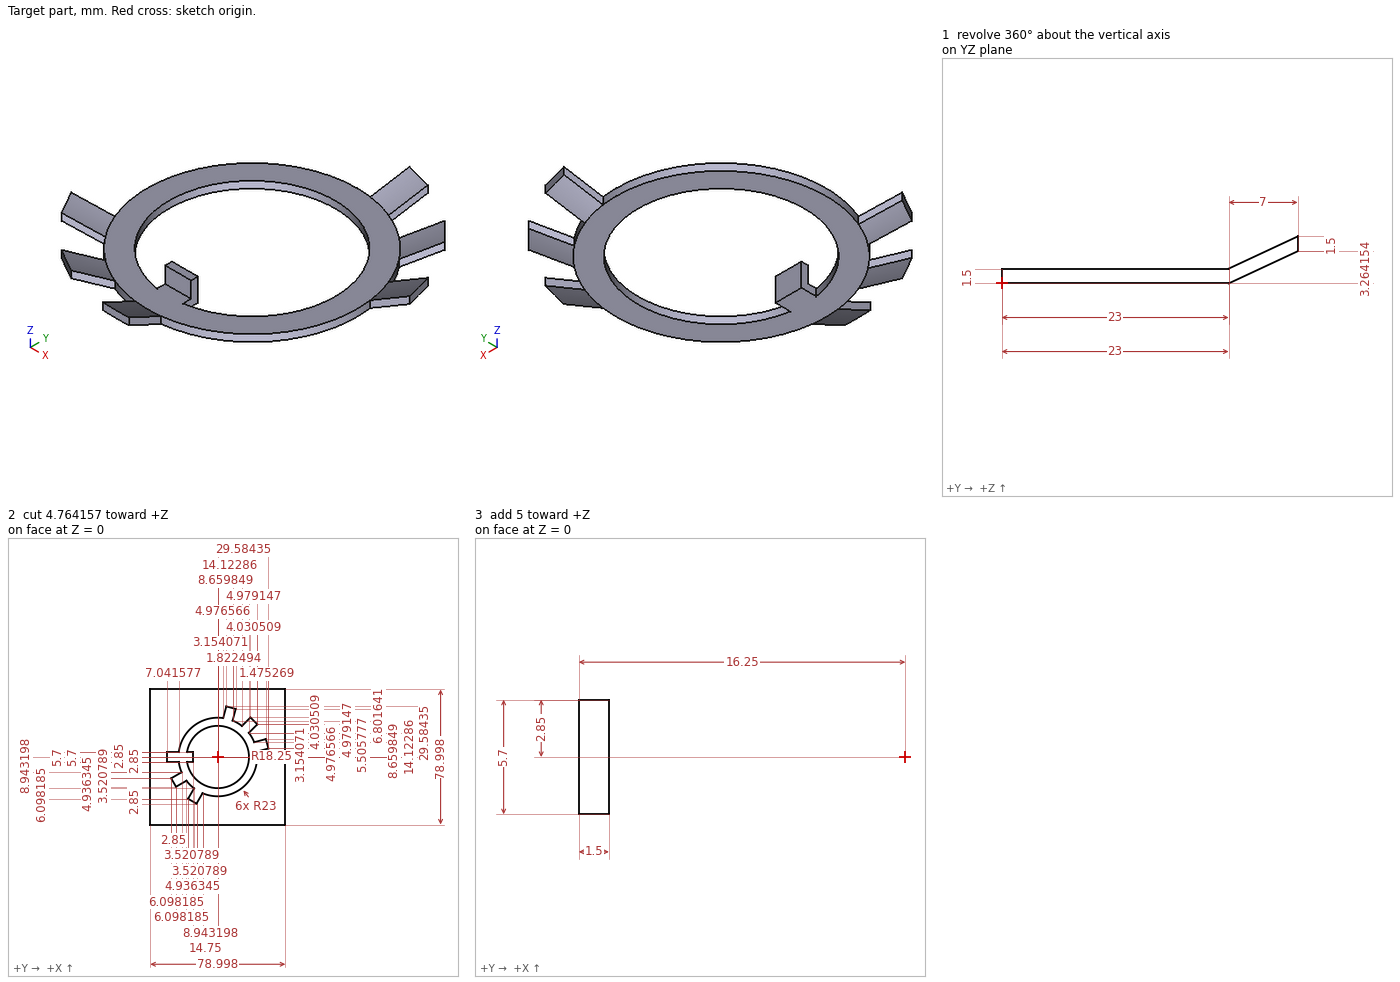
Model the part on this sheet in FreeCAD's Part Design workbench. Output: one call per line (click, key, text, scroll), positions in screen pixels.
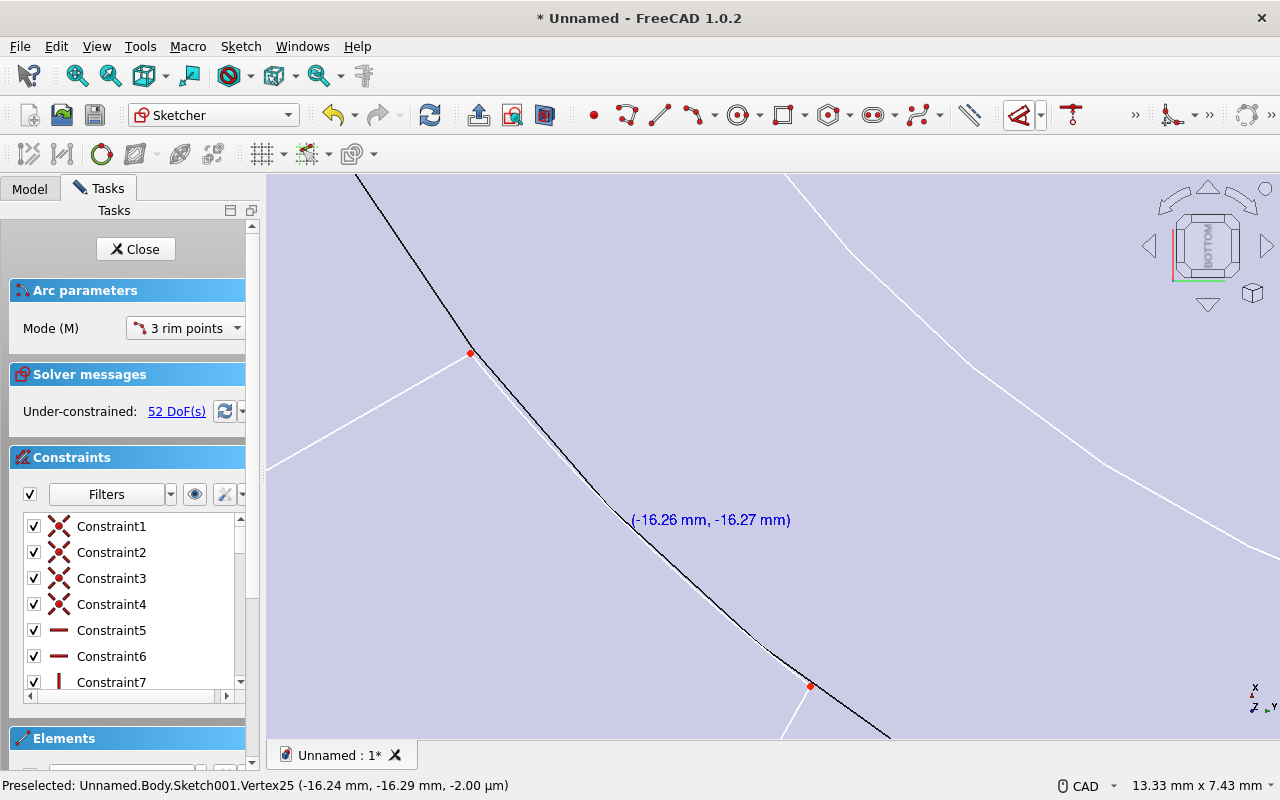
scroll(629, 532, down, 14)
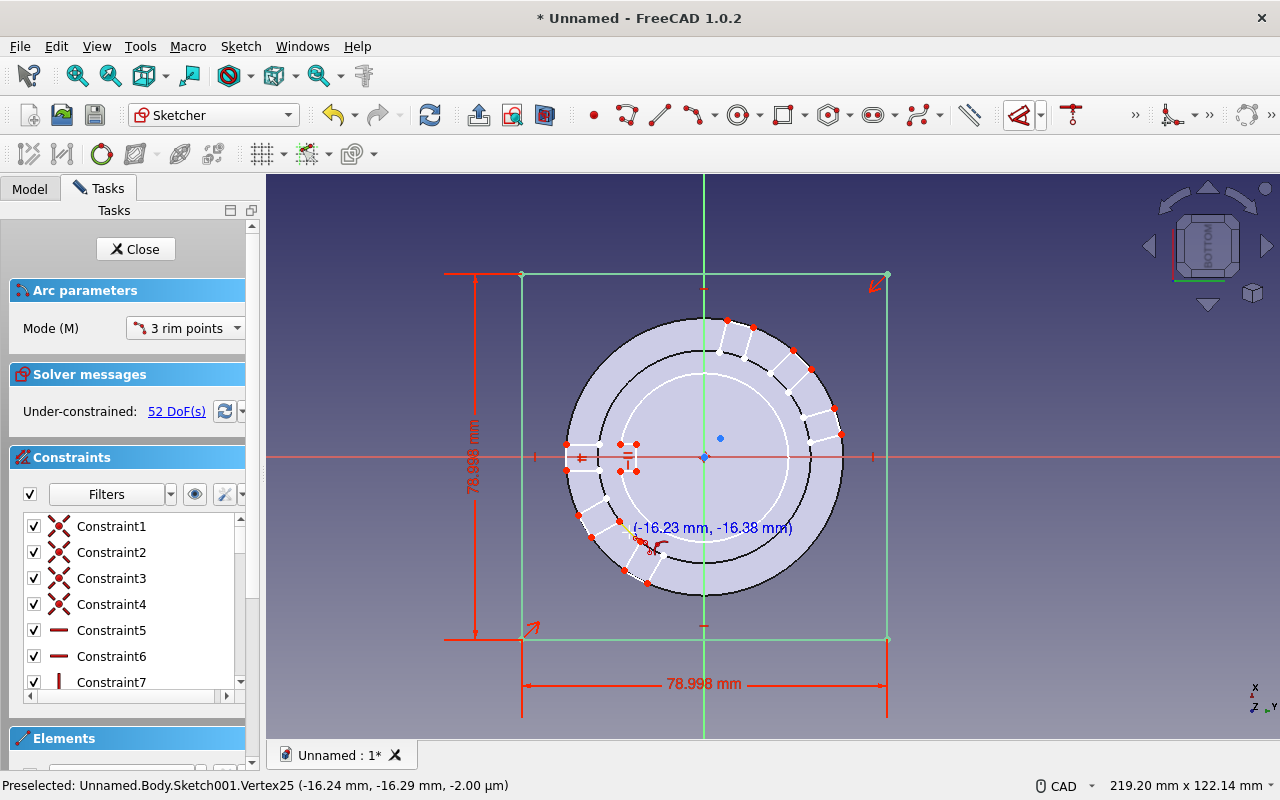
click(663, 556)
click(810, 443)
click(769, 541)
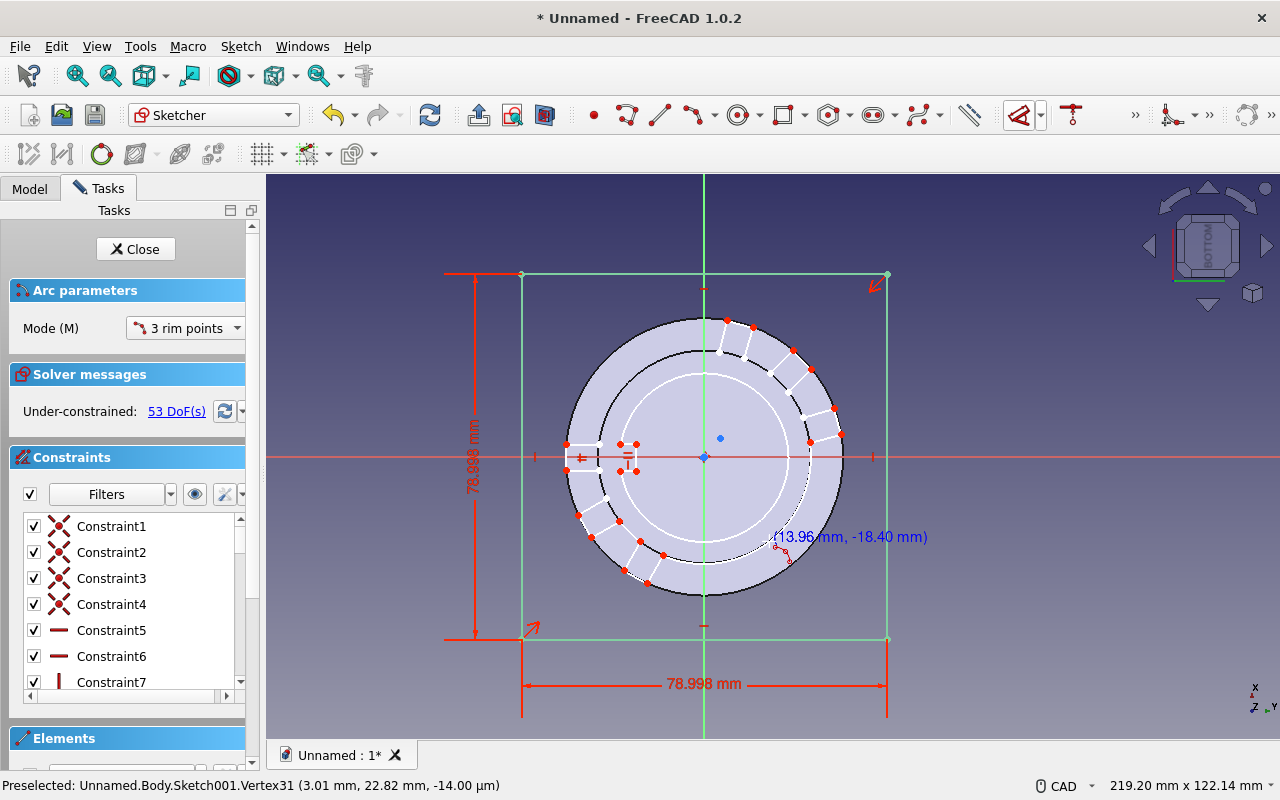
click(803, 418)
click(788, 393)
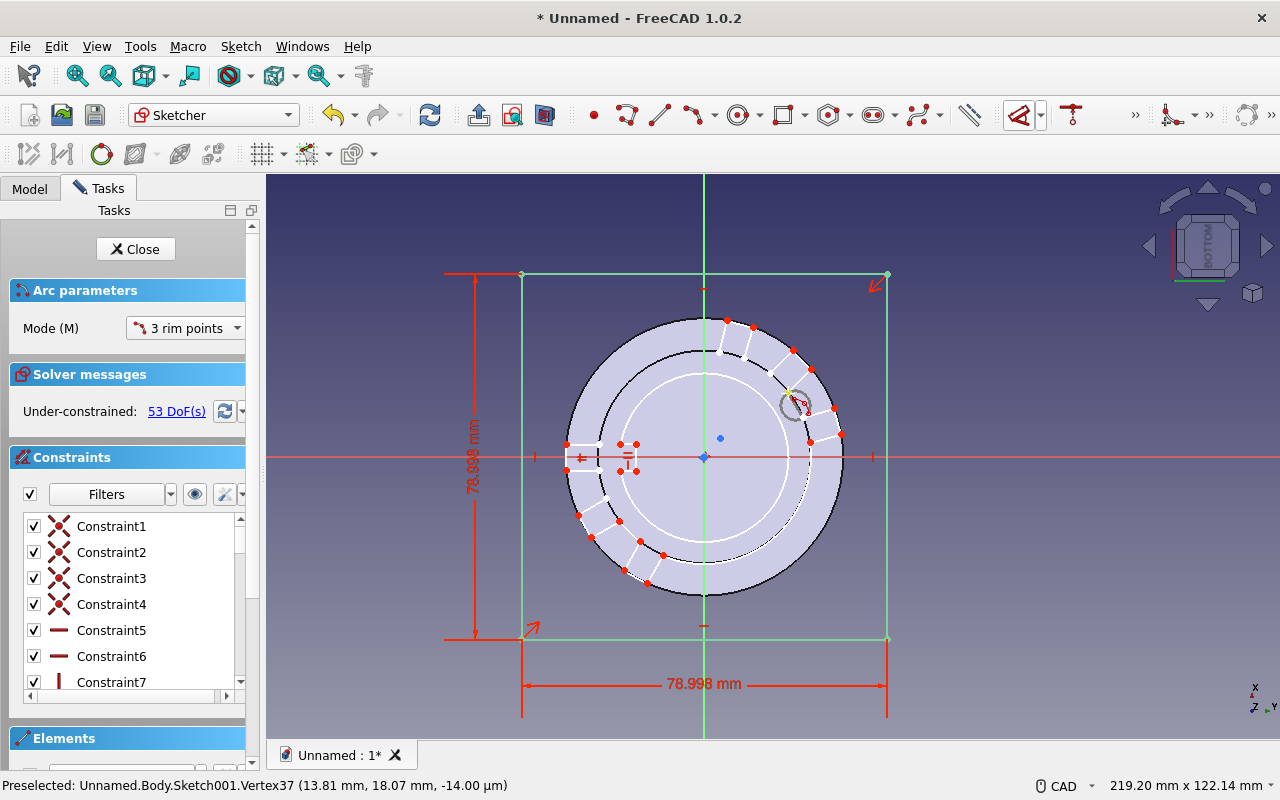
scroll(797, 404, up, 14)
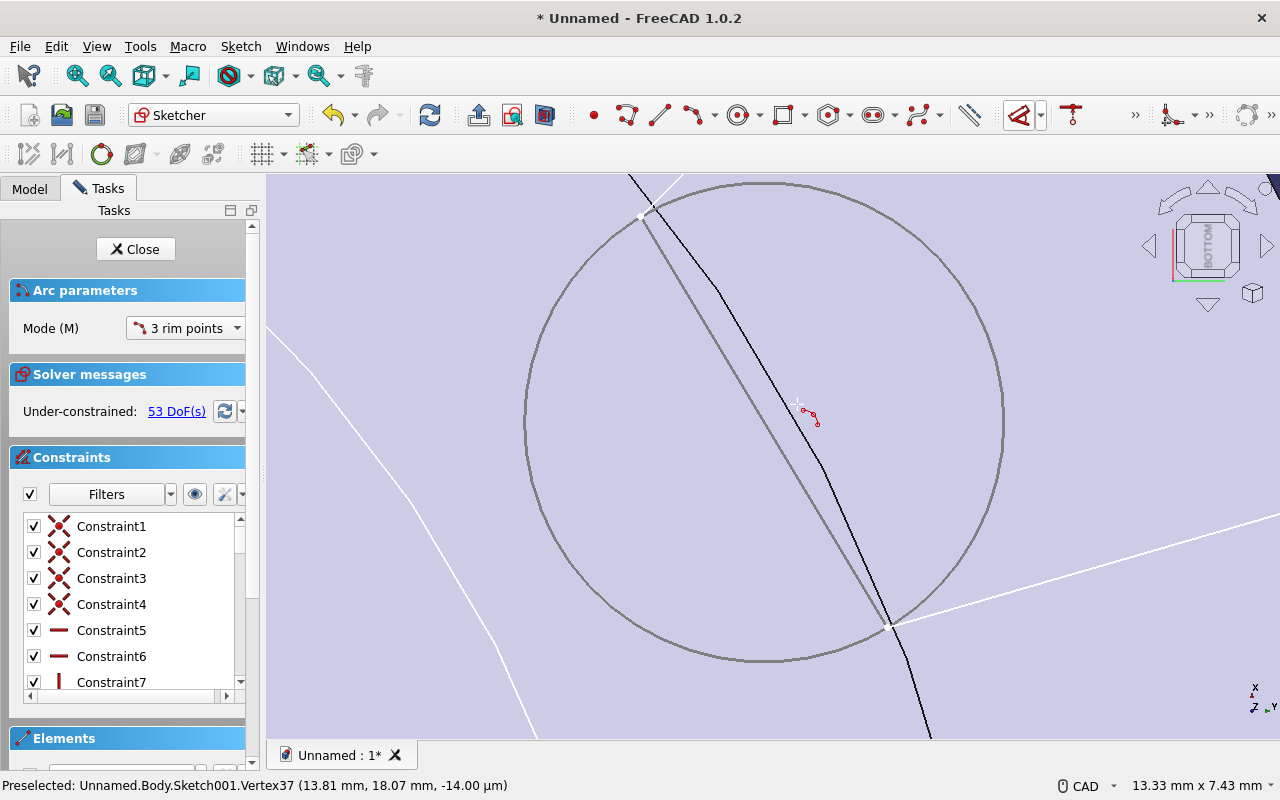
click(782, 393)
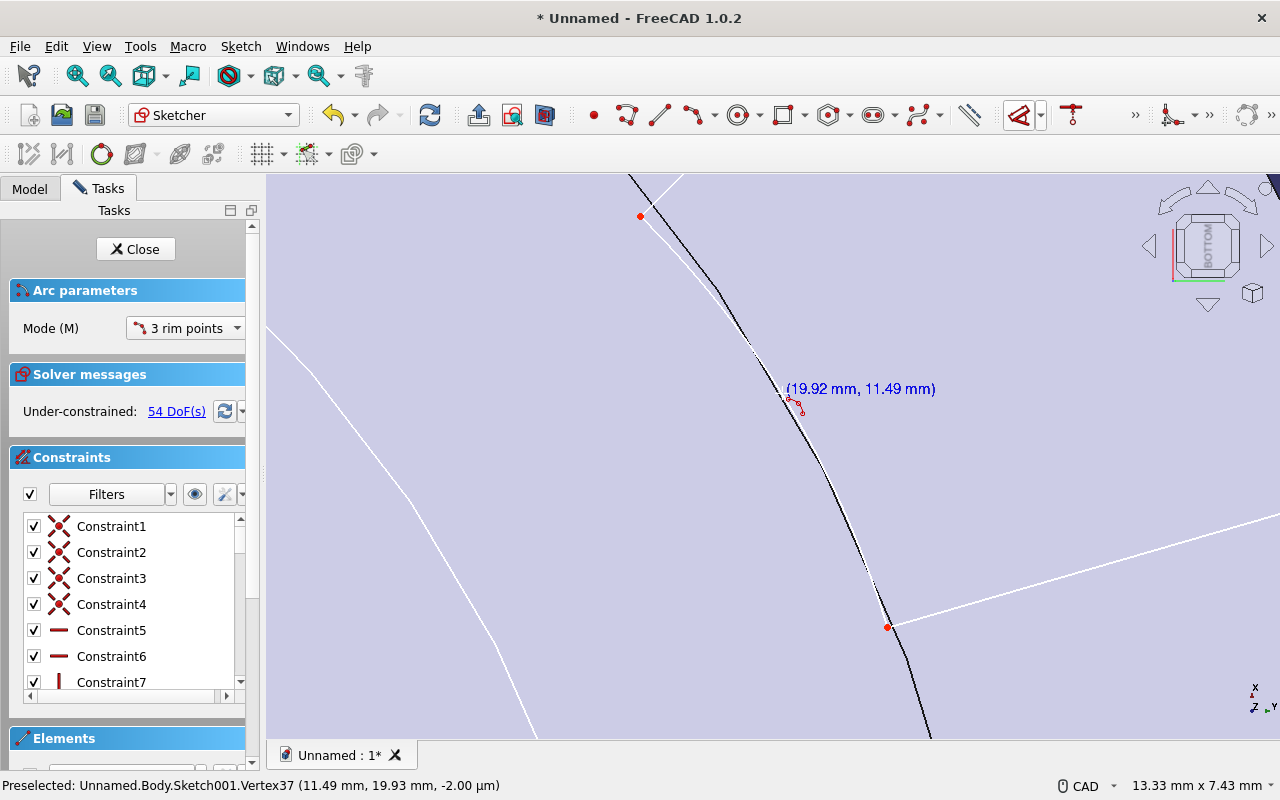
scroll(798, 404, down, 14)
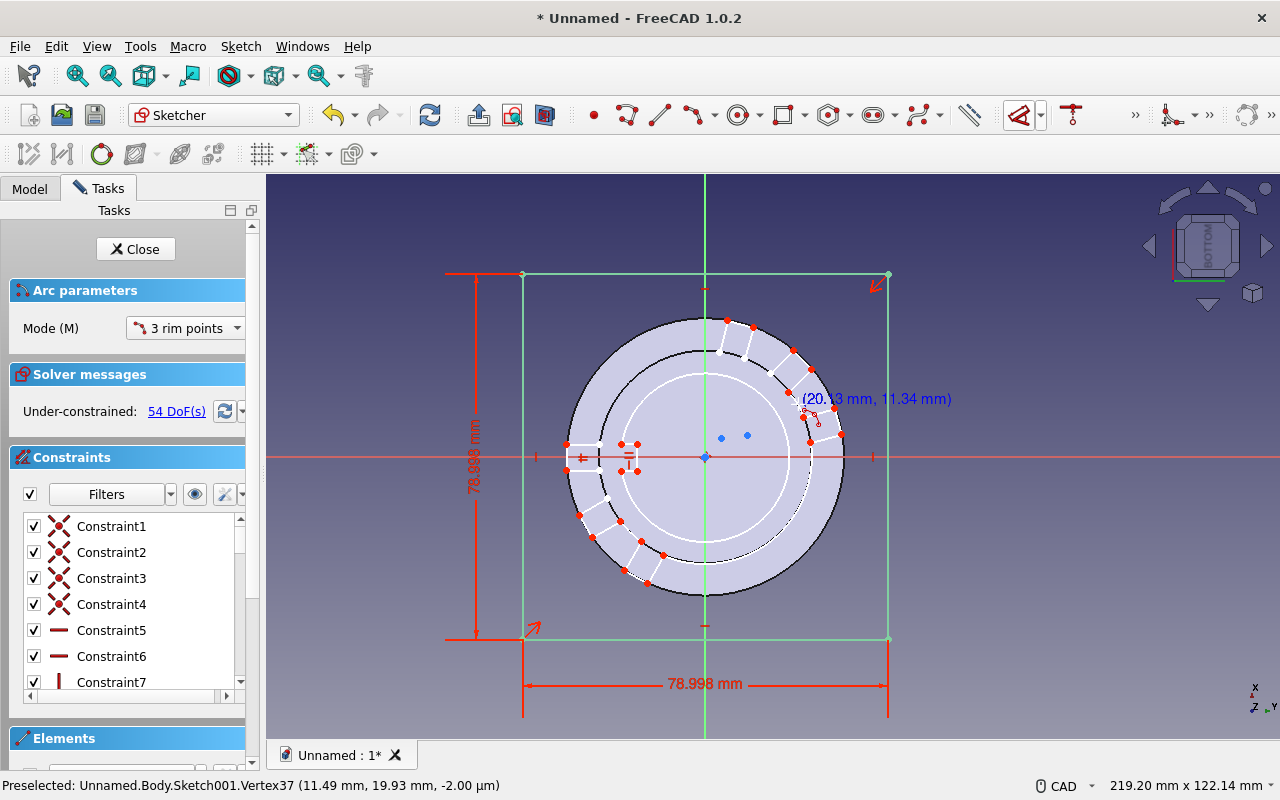
click(771, 374)
click(745, 359)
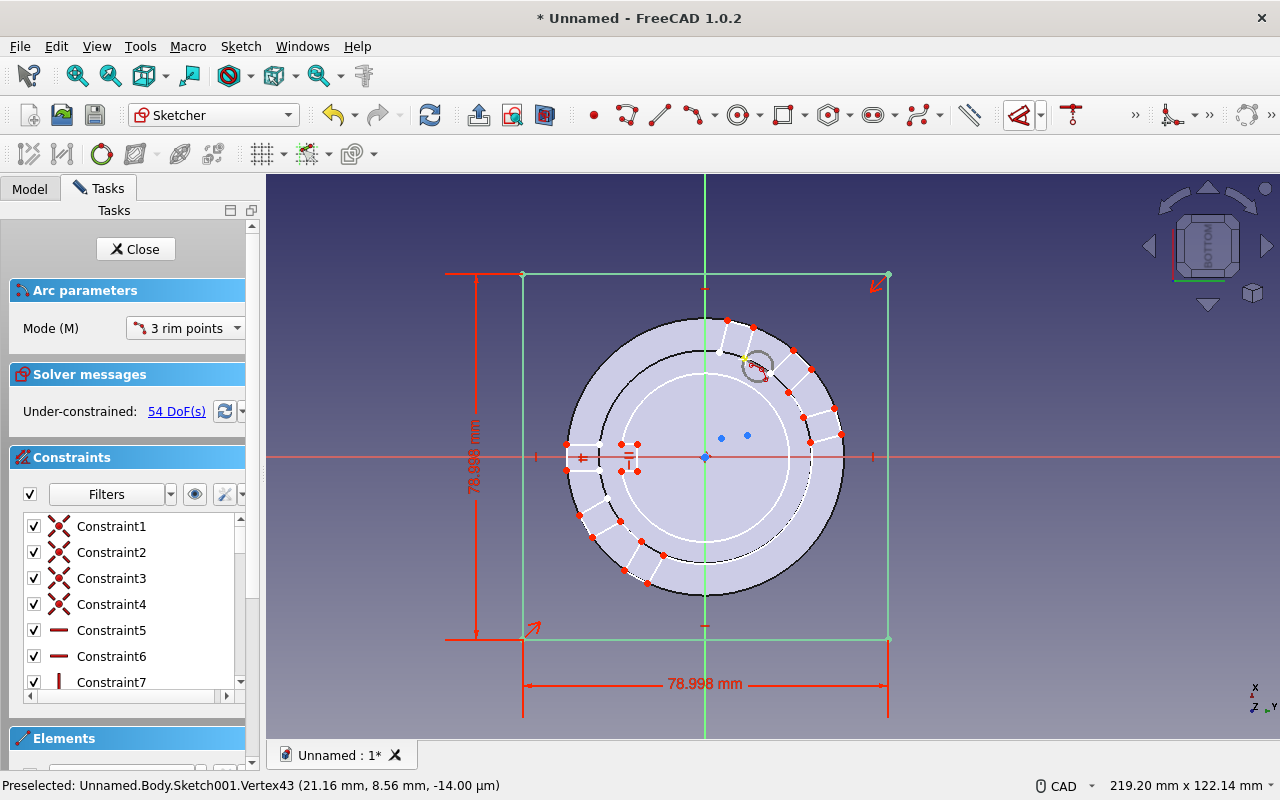
scroll(759, 365, up, 14)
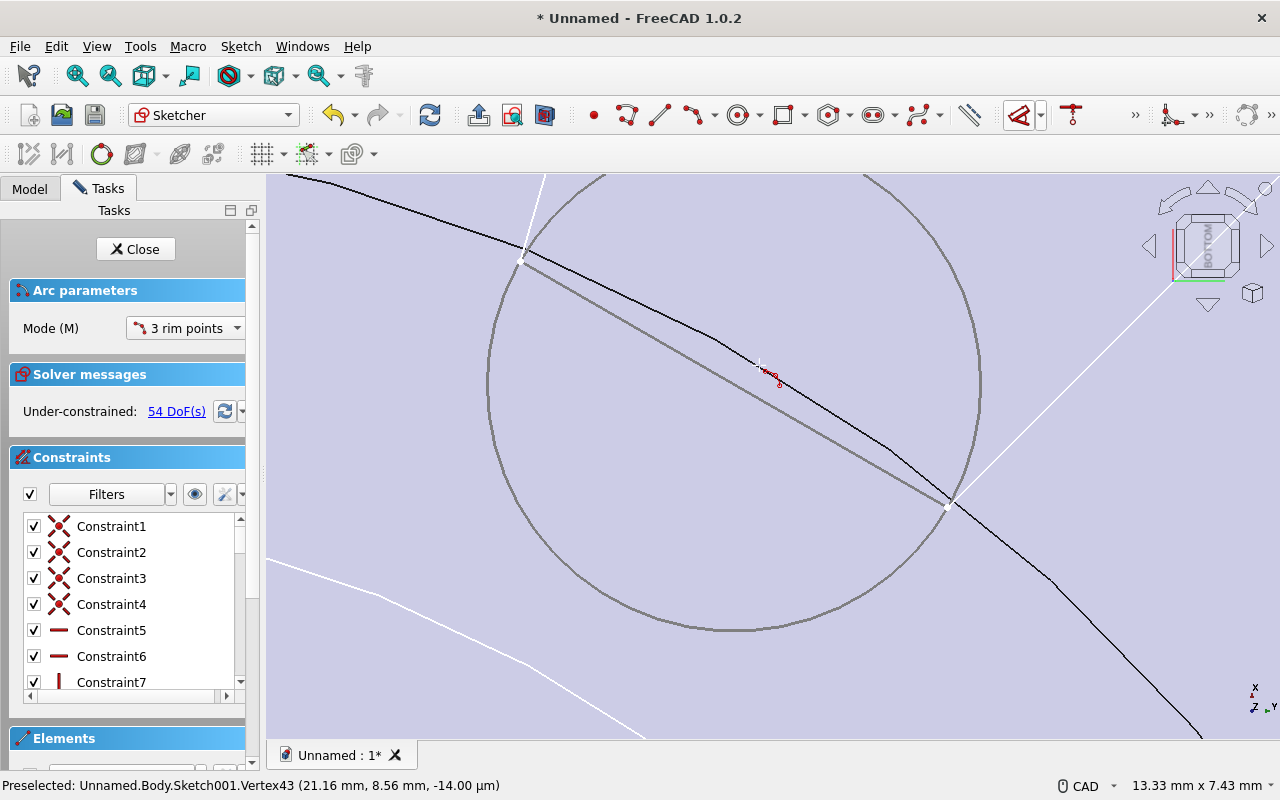
click(744, 356)